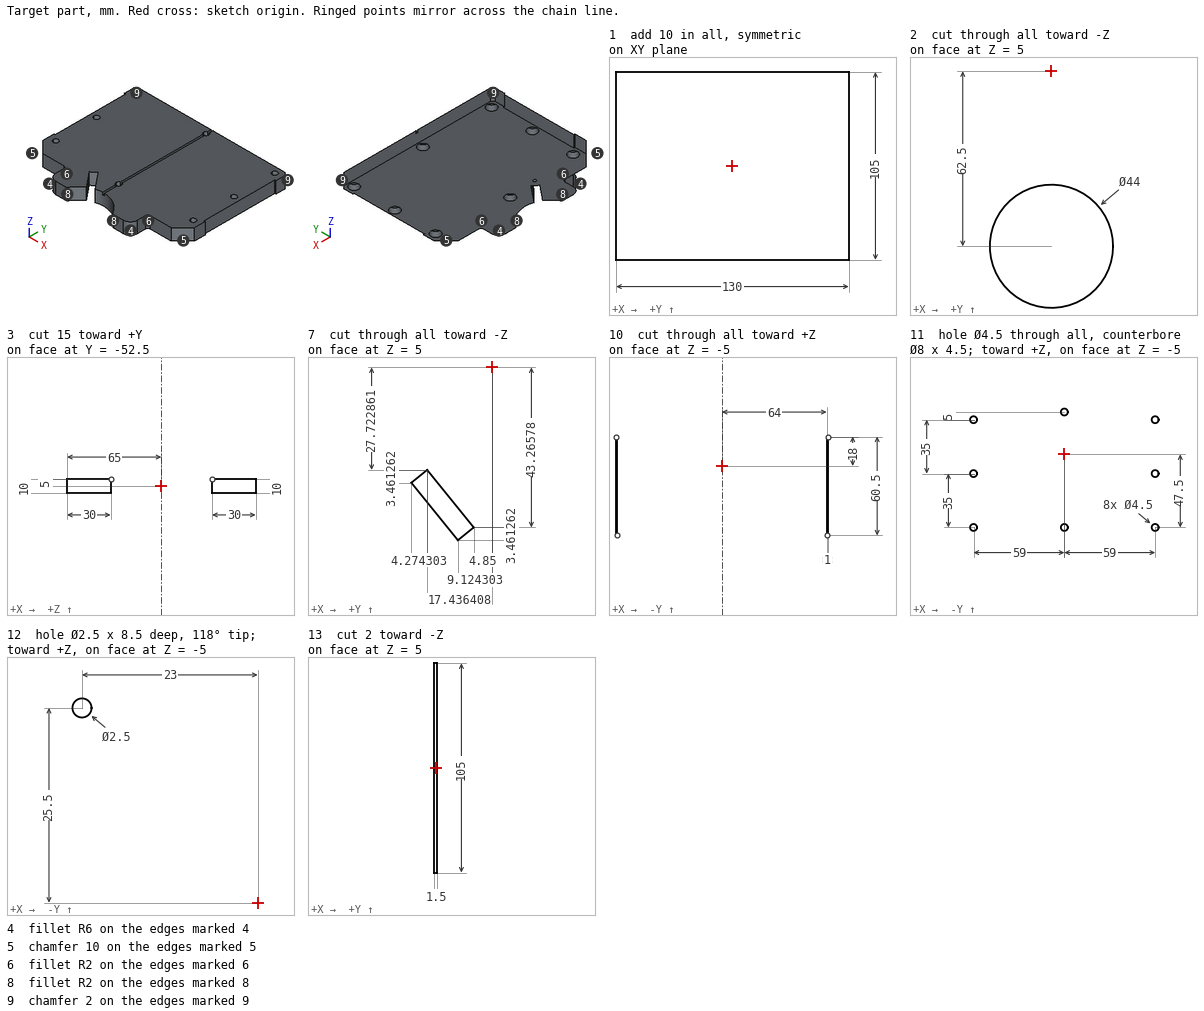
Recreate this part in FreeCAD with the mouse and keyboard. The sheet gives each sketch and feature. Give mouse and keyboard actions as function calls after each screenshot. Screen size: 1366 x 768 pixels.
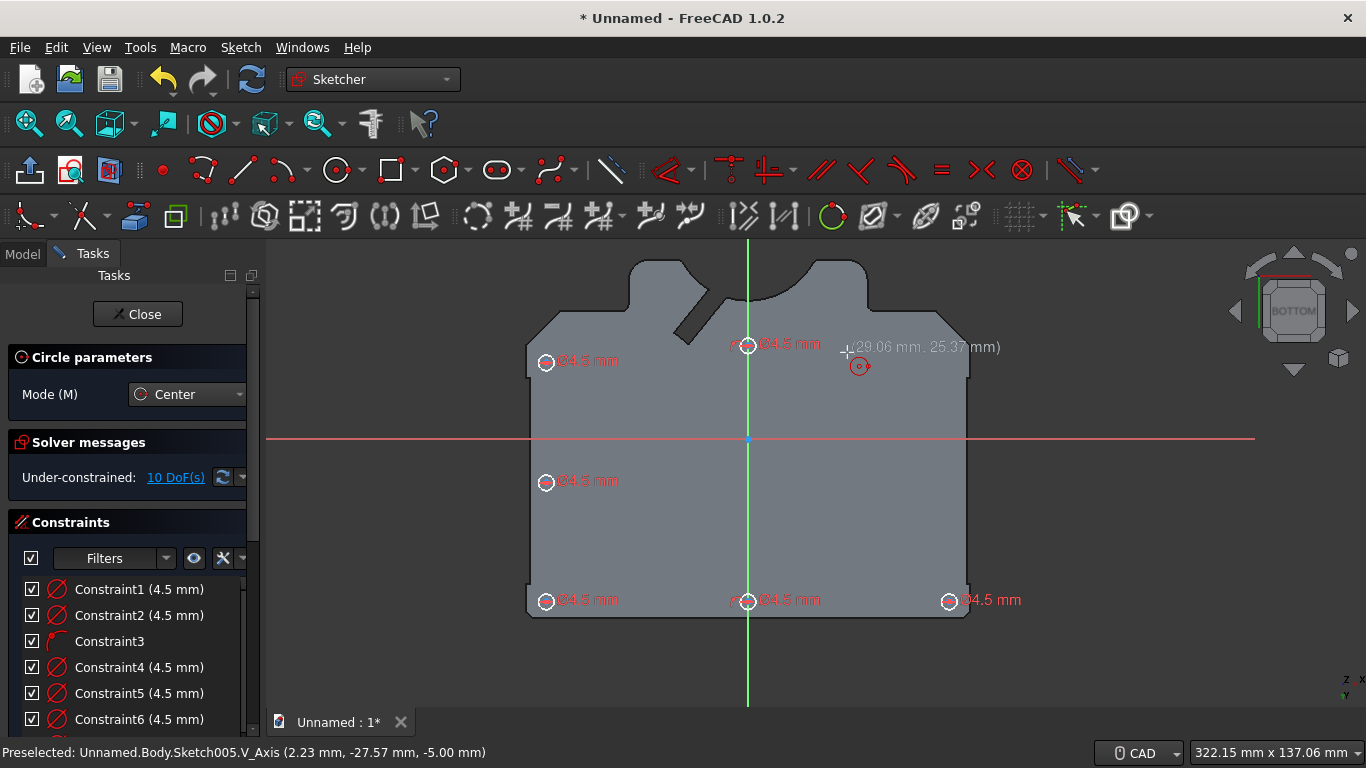
click(950, 362)
move(955, 357)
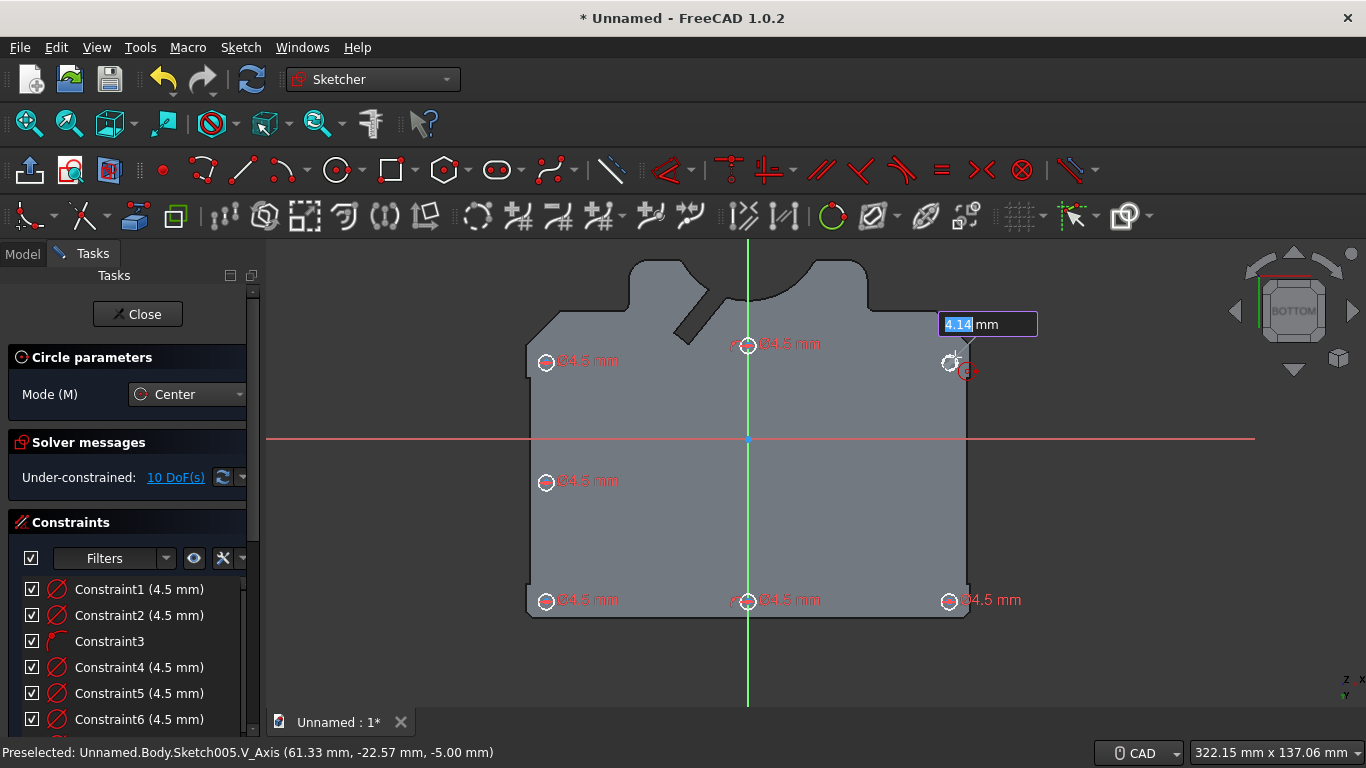
text(4.5)
key(Return)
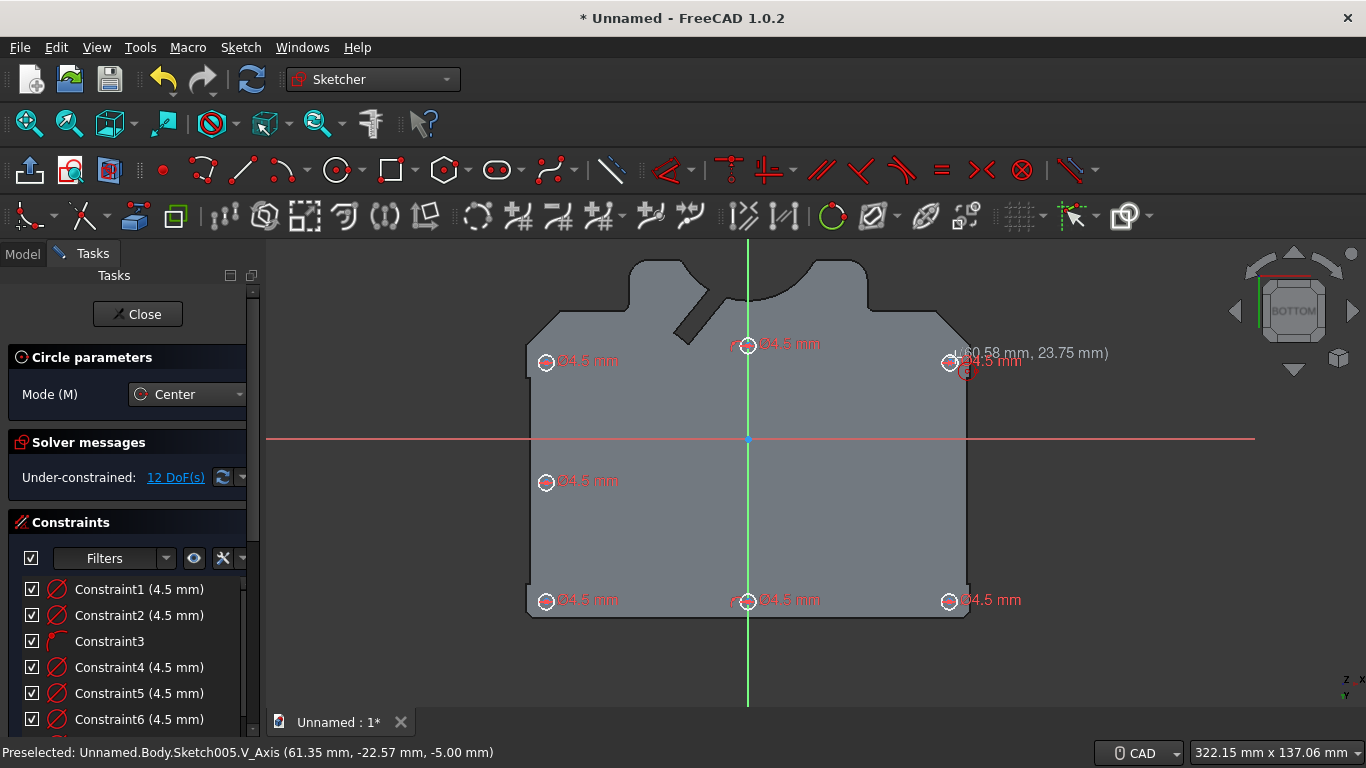
scroll(950, 482, up, 6)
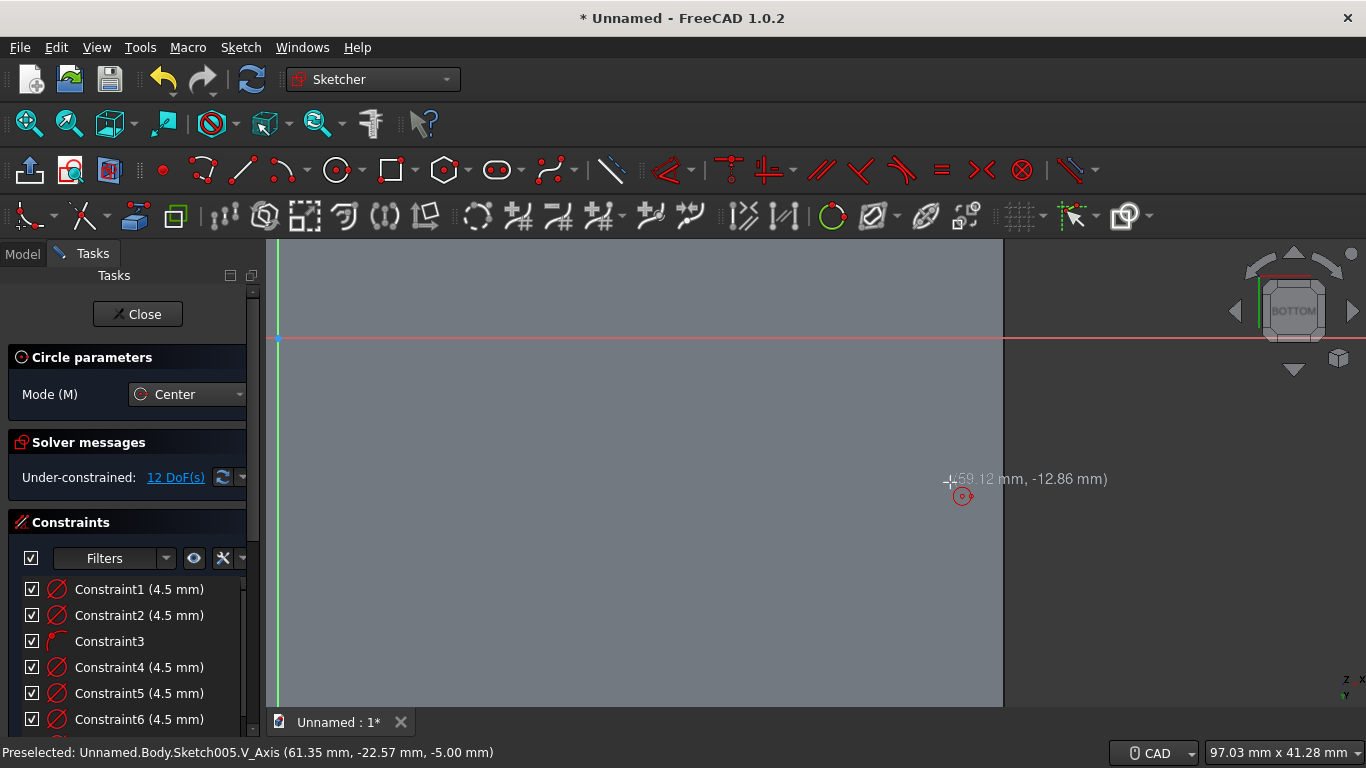
scroll(950, 482, down, 6)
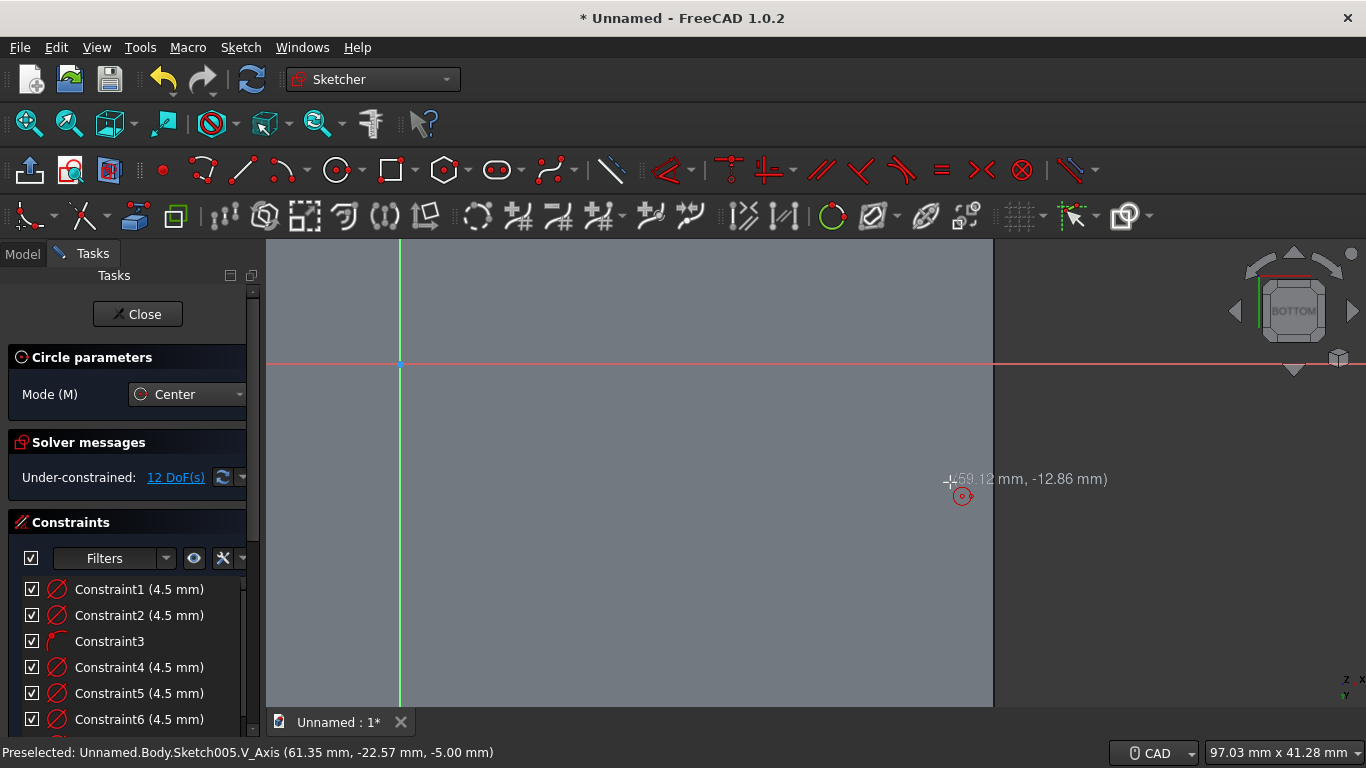
click(950, 482)
move(955, 476)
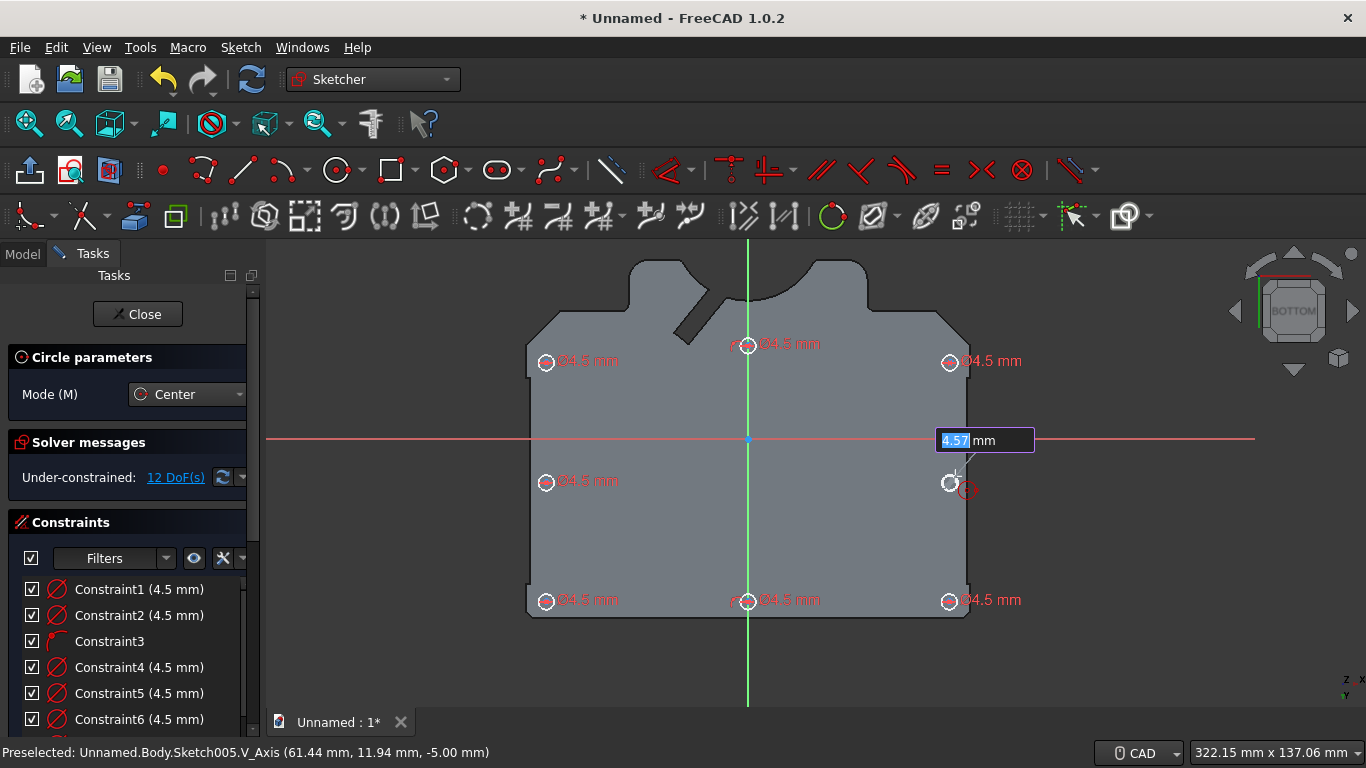
text(4.5)
key(Return)
key(Escape)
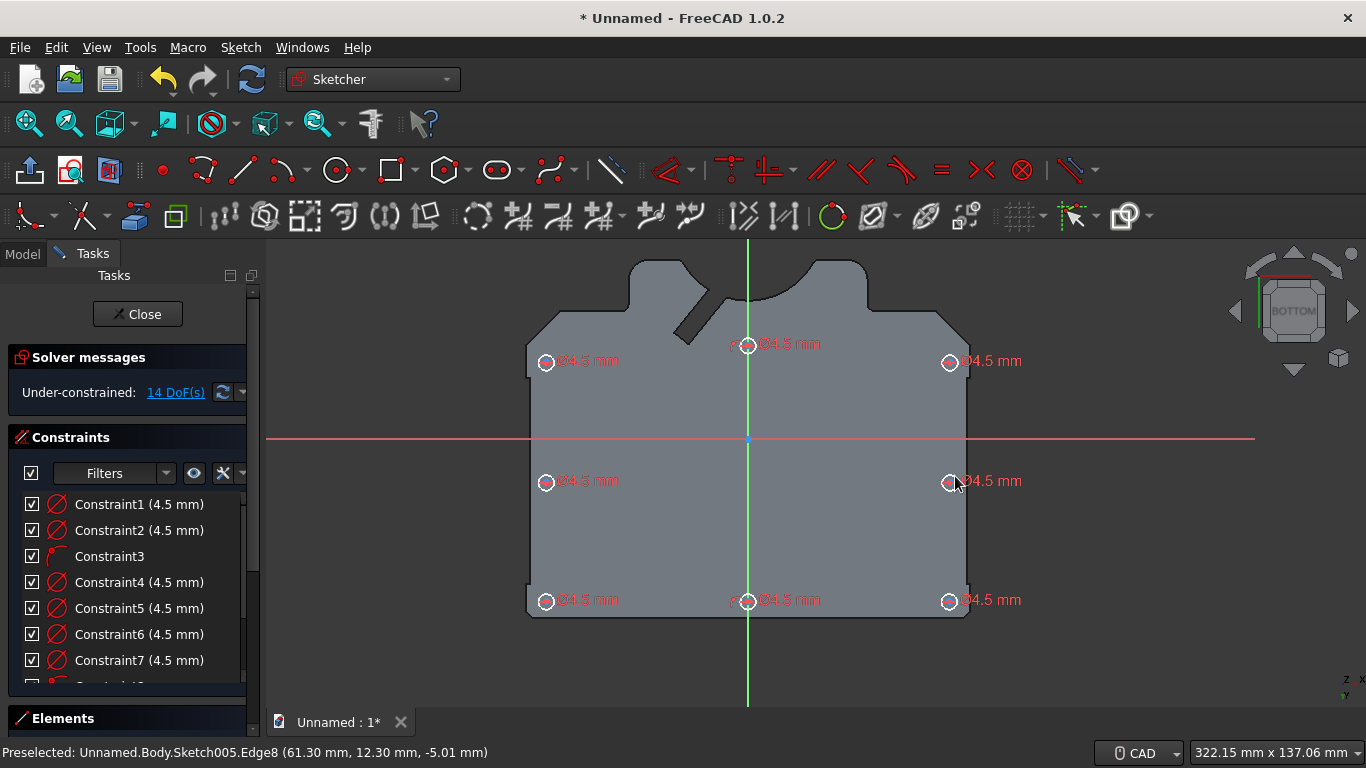
click(949, 602)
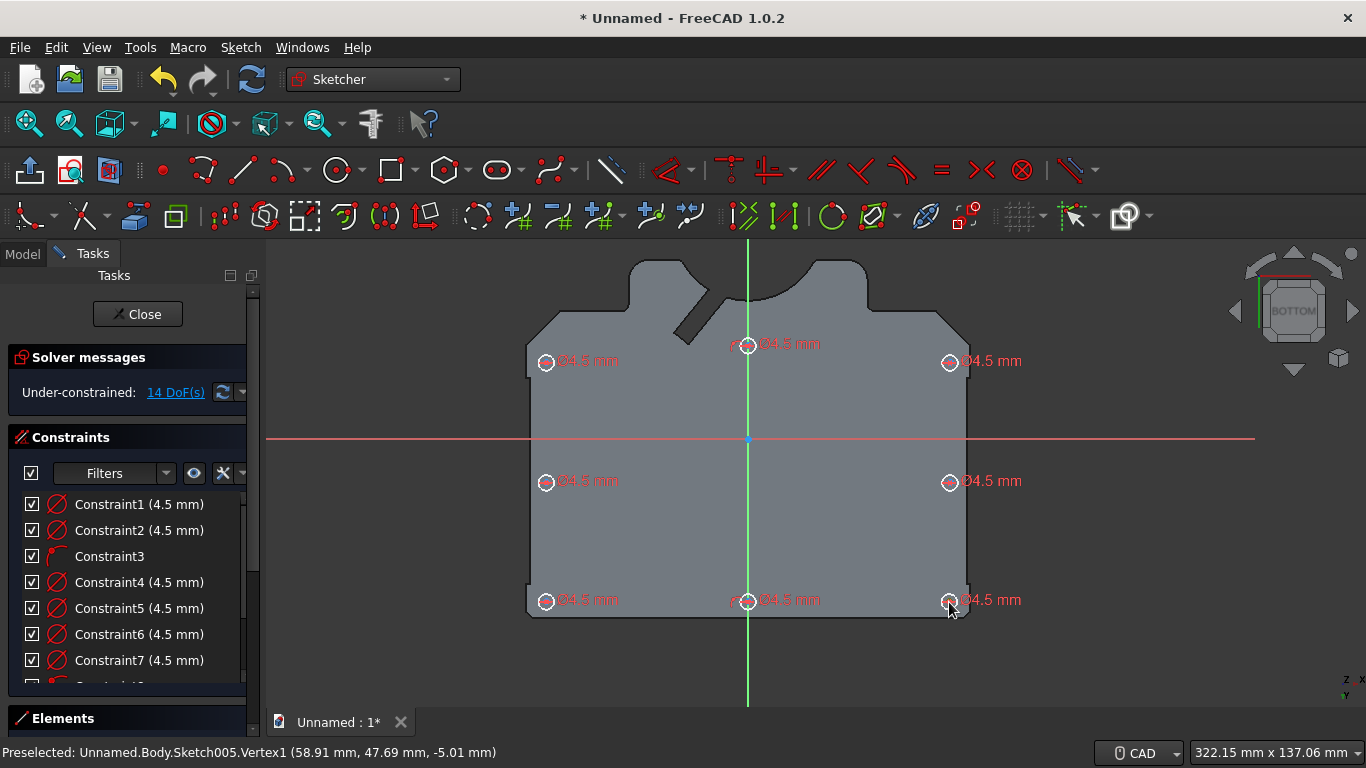
click(748, 602)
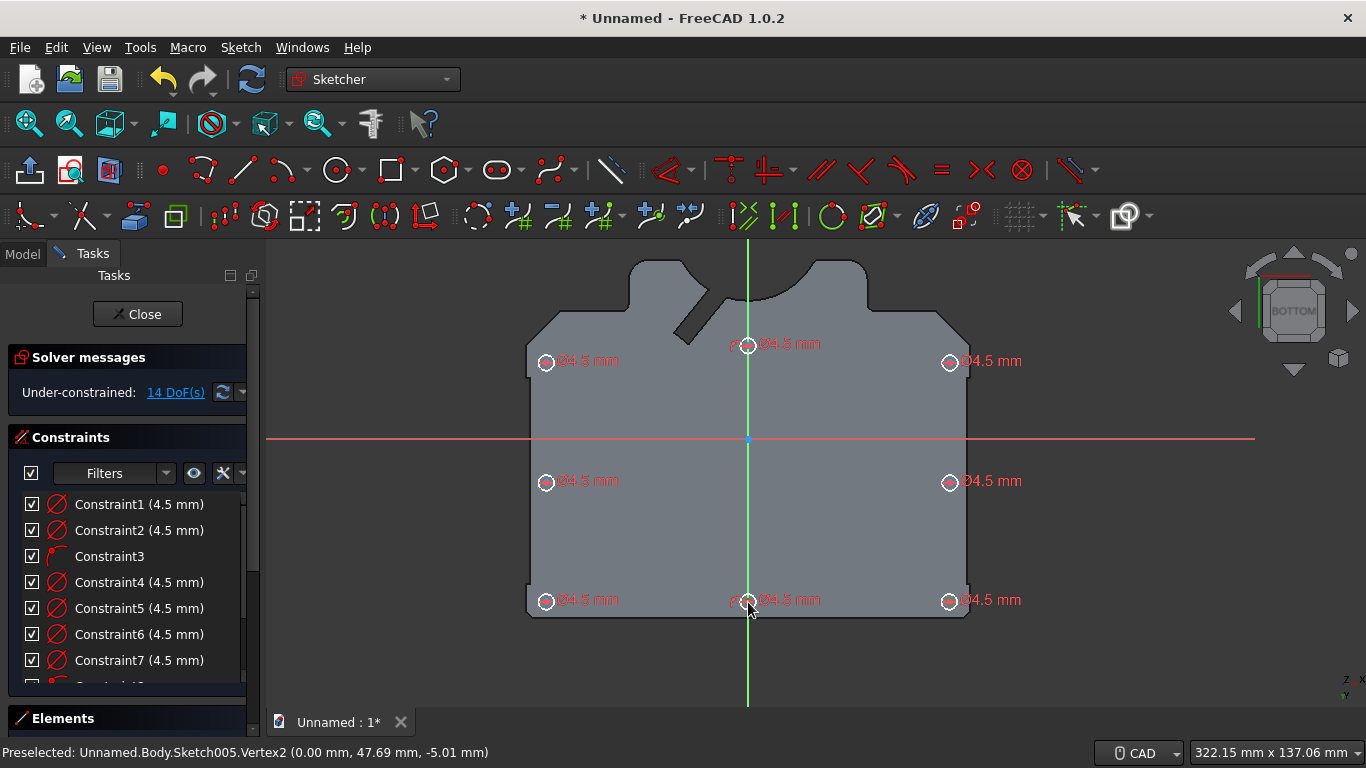
key(h)